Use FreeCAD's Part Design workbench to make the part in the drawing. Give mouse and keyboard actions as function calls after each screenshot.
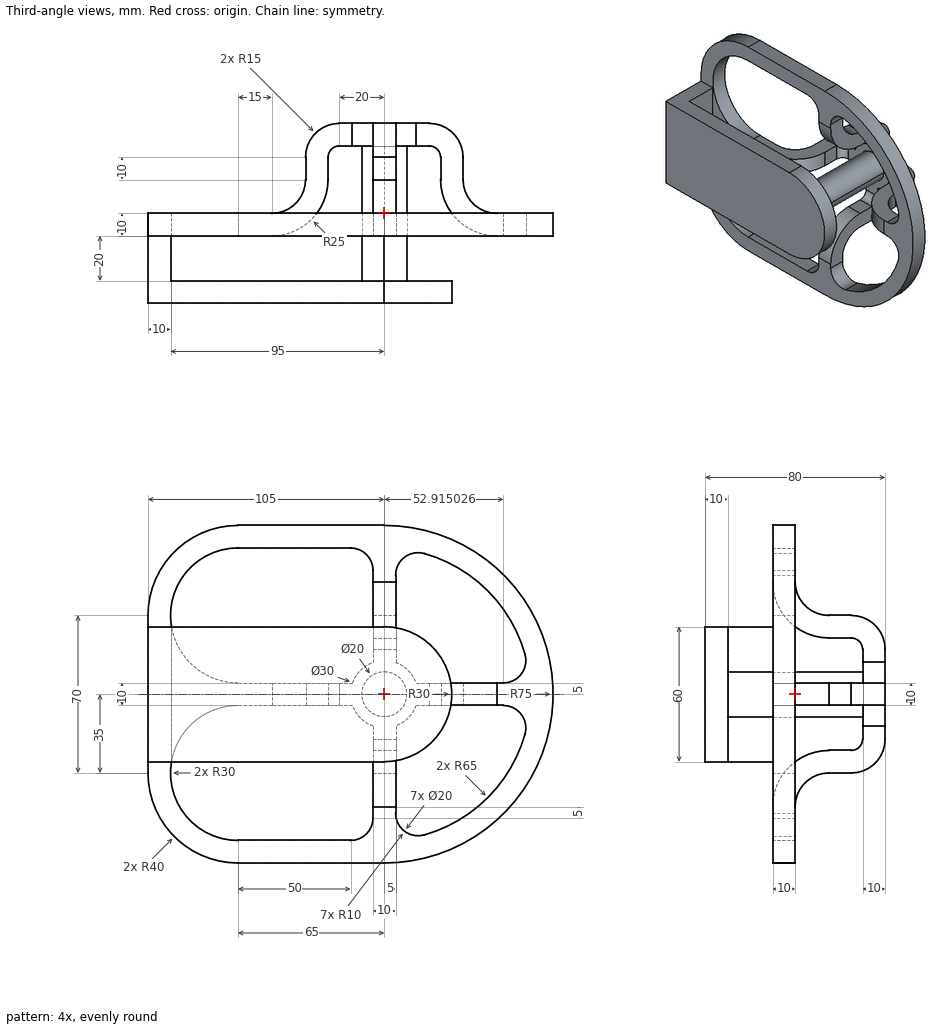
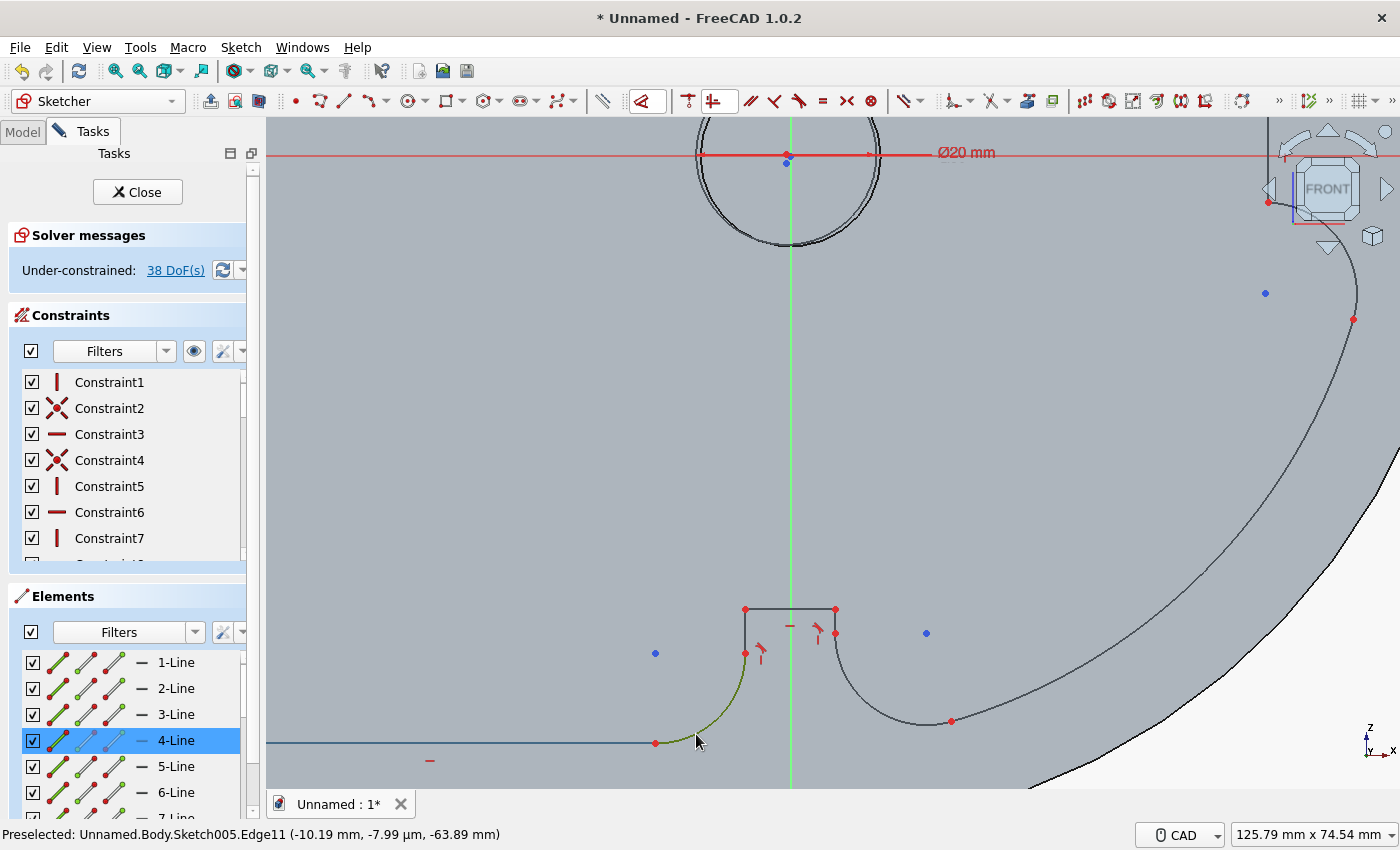
click(800, 102)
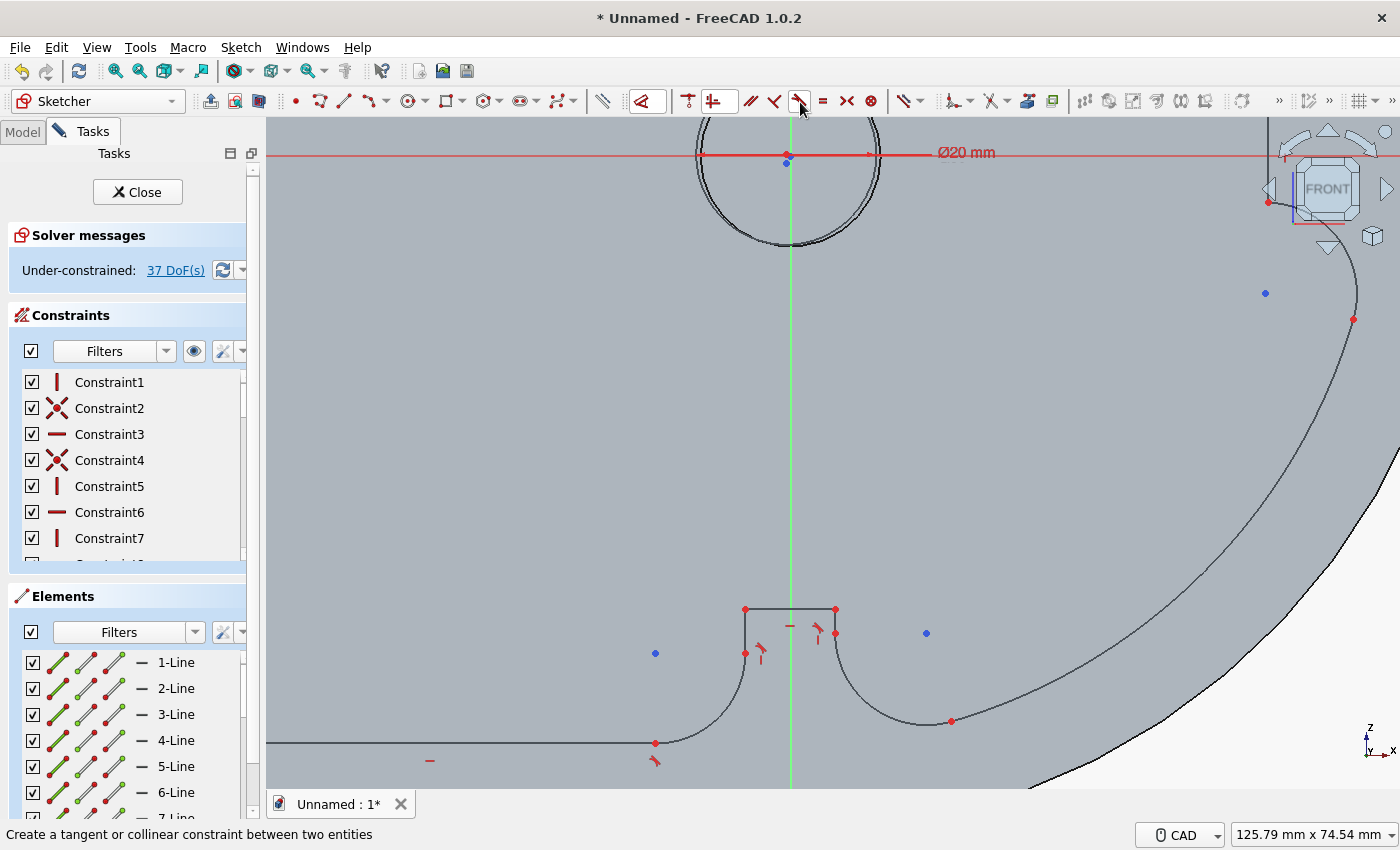
click(520, 743)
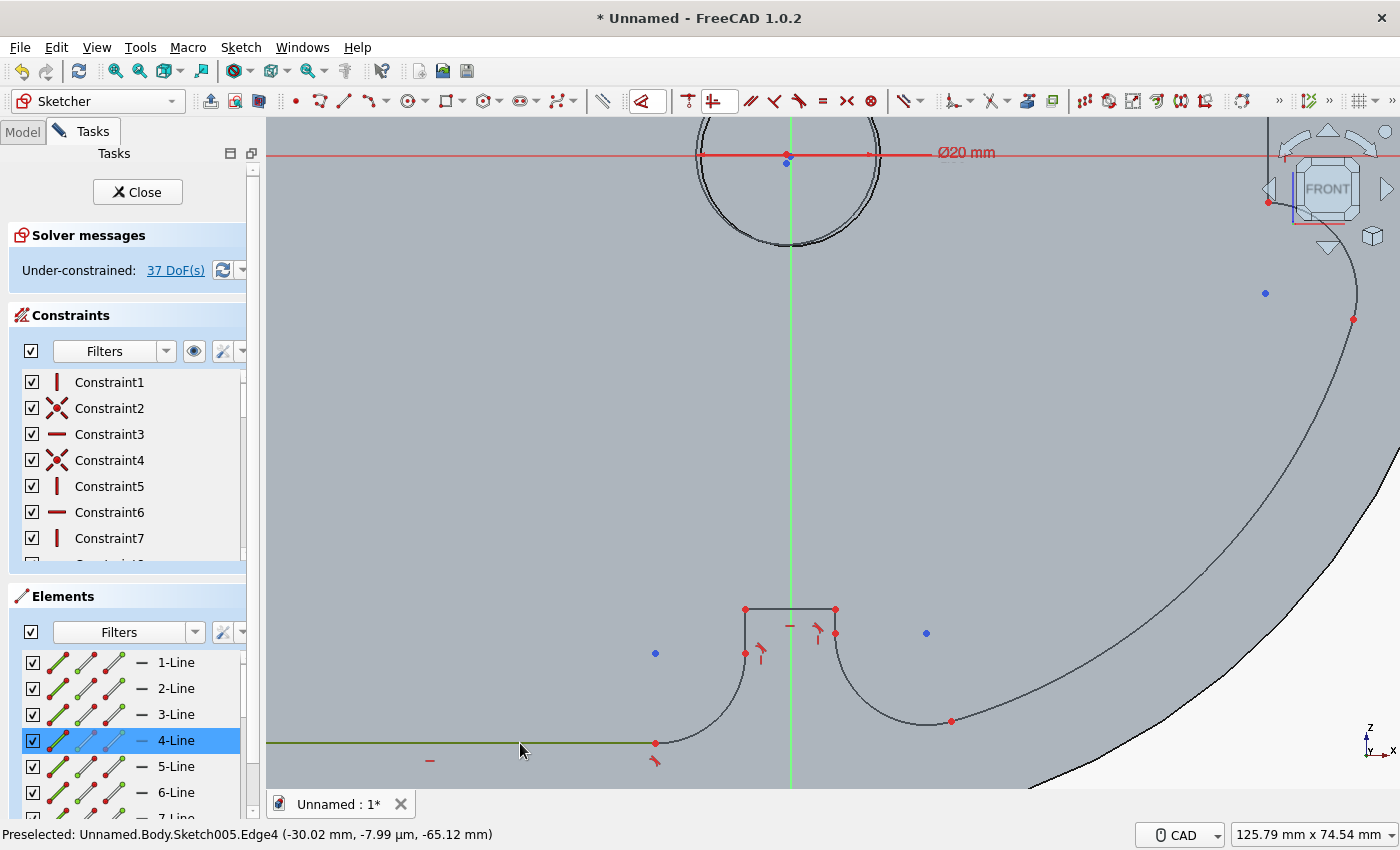
scroll(834, 626, down, 5)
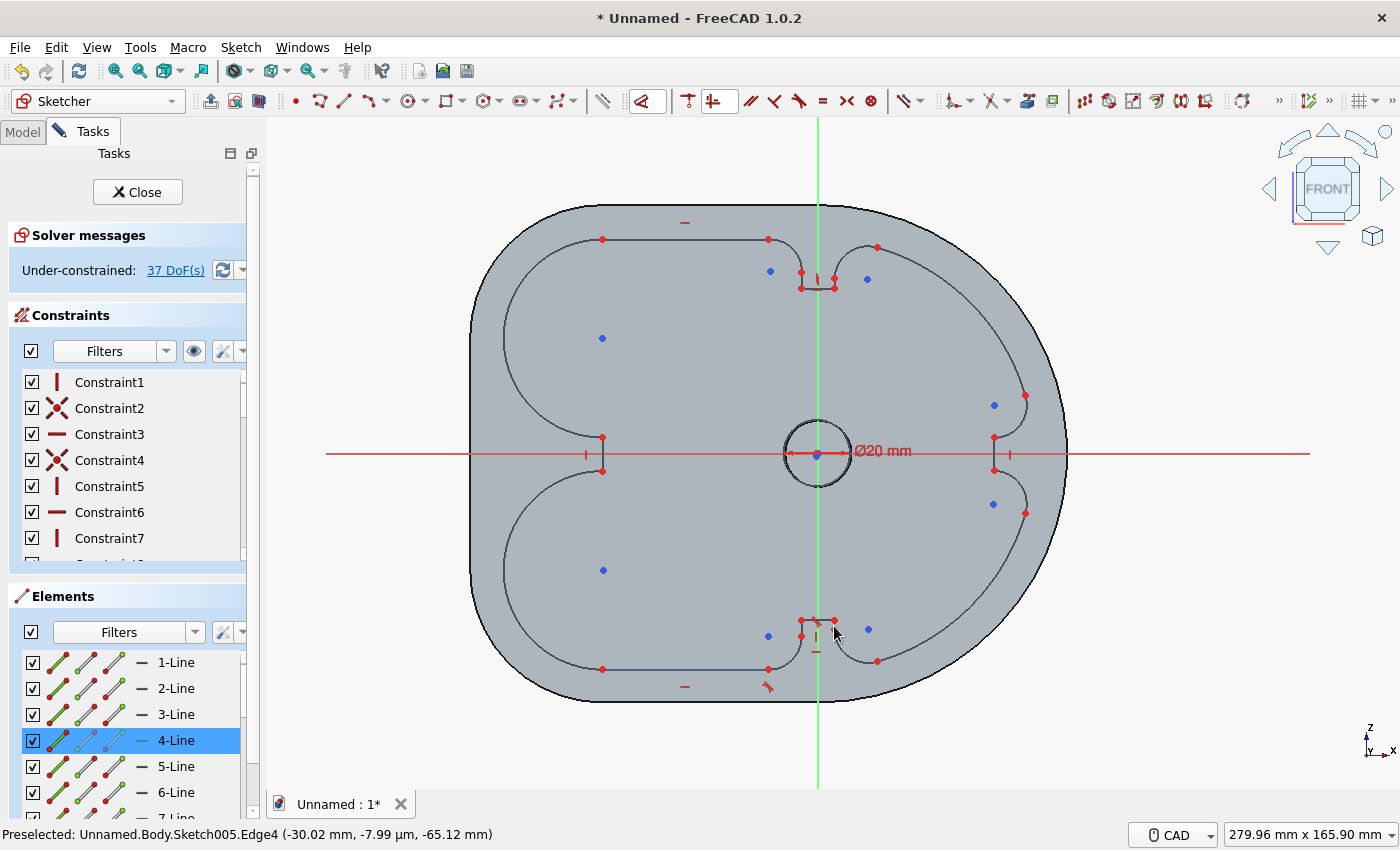
click(523, 512)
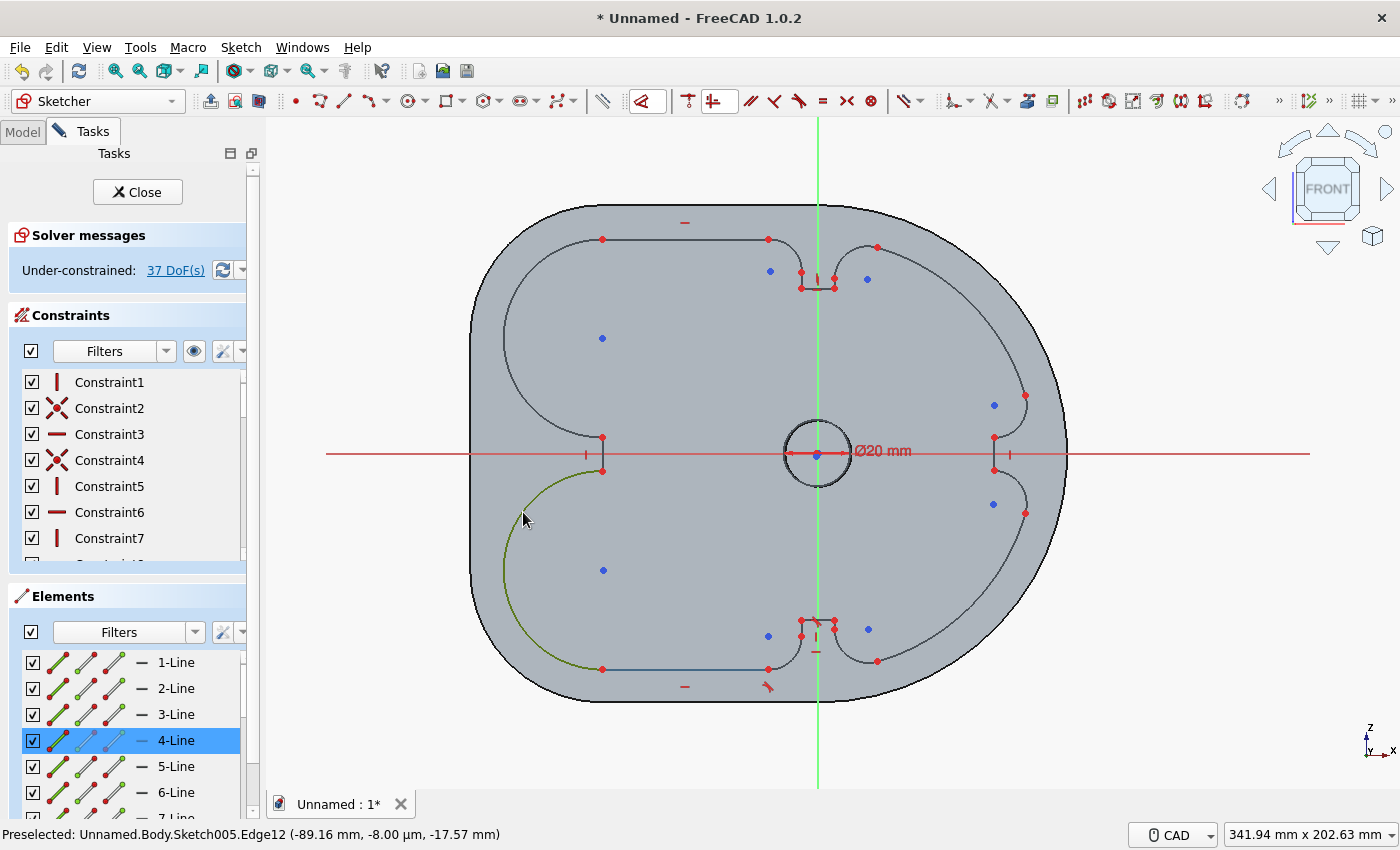
click(800, 102)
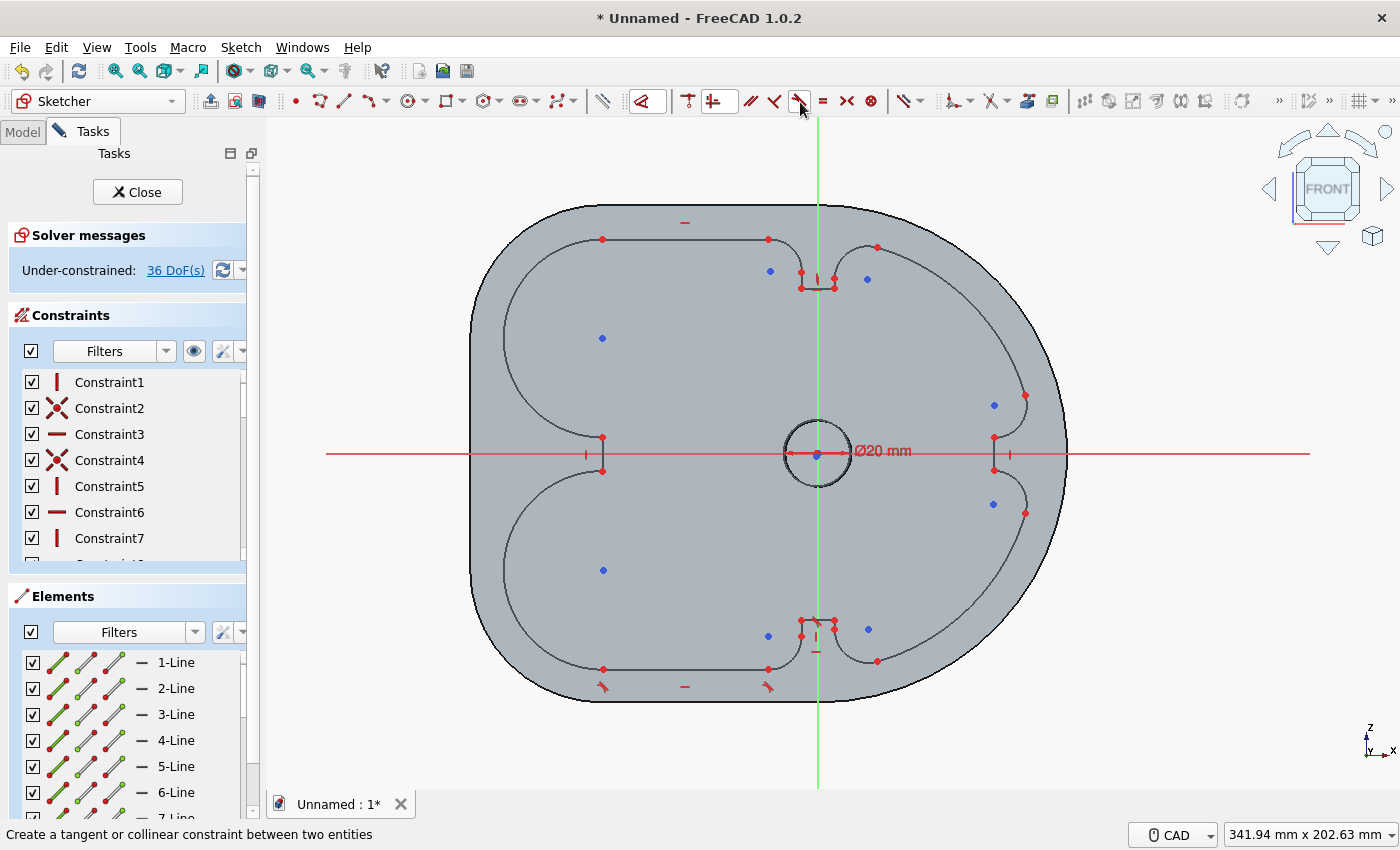
click(653, 240)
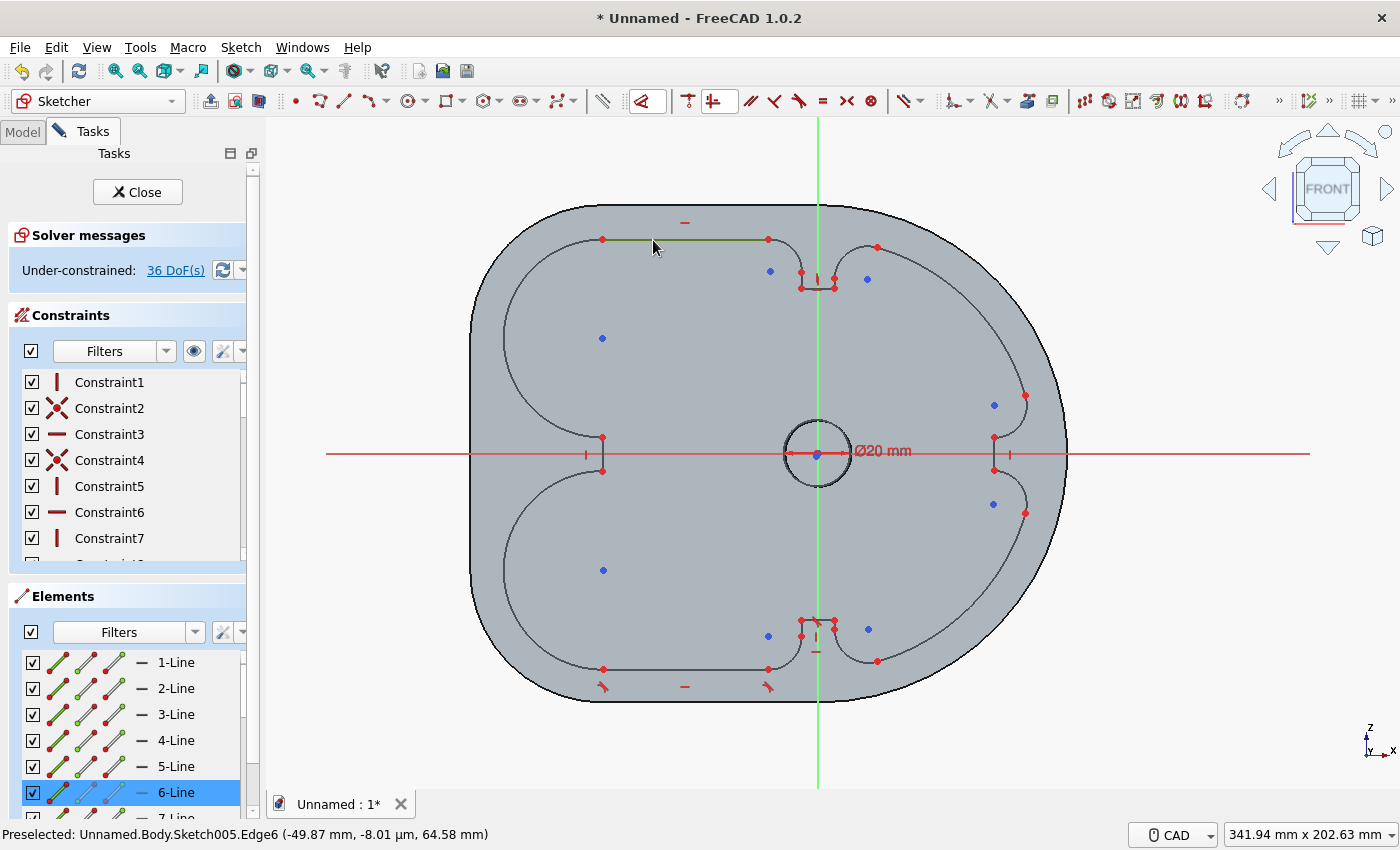
click(523, 280)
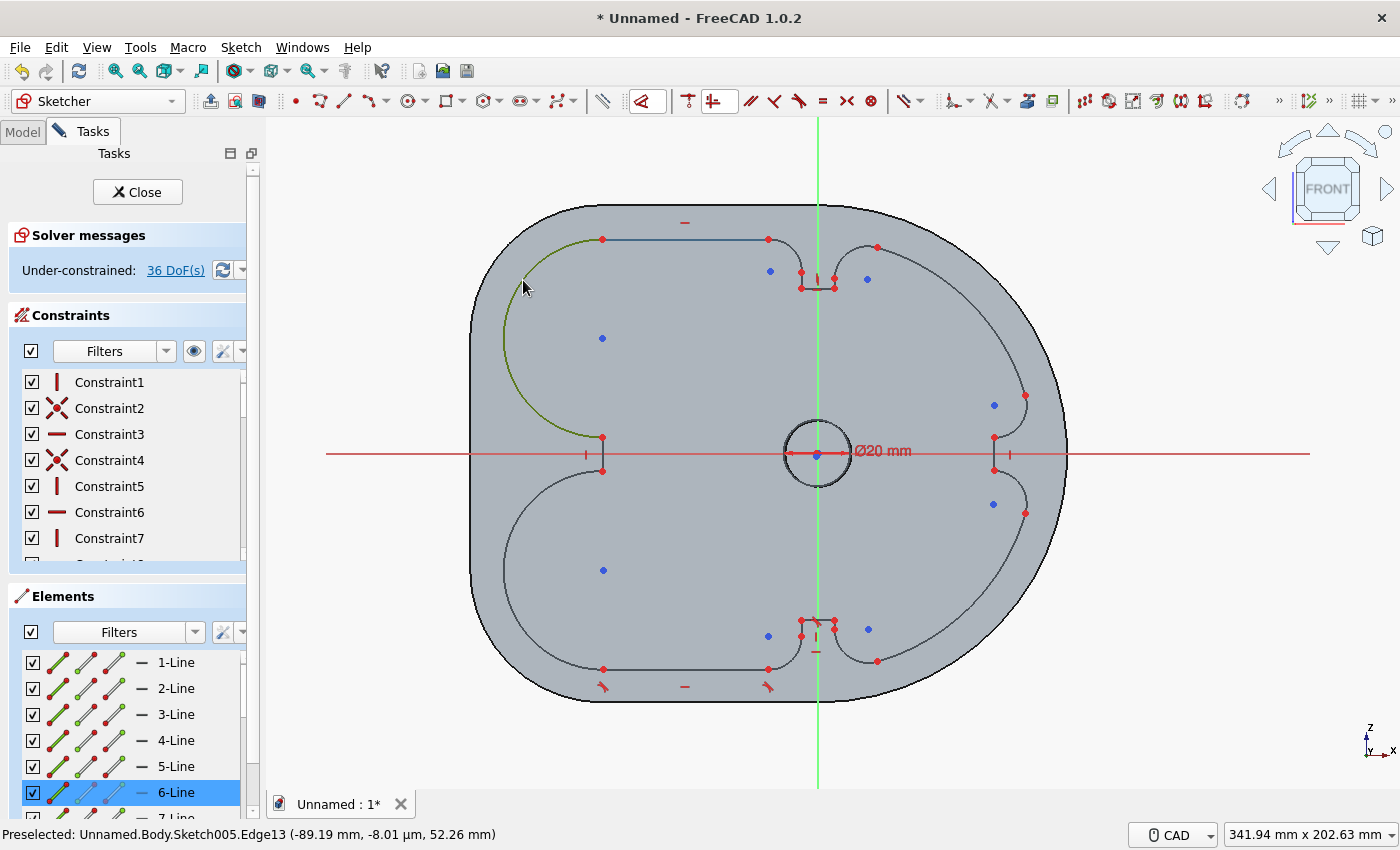
click(800, 102)